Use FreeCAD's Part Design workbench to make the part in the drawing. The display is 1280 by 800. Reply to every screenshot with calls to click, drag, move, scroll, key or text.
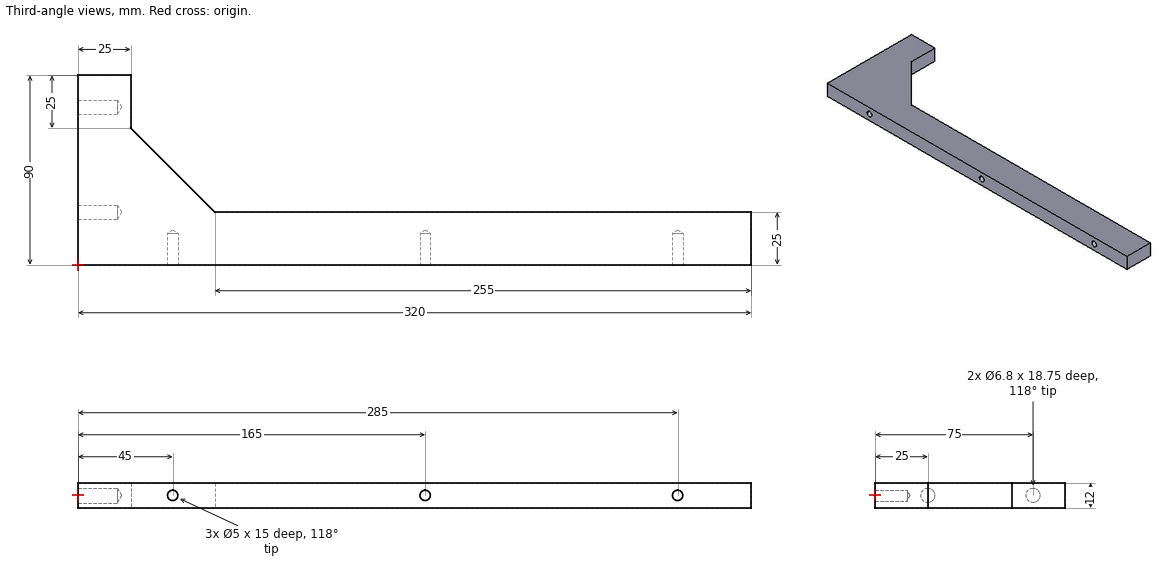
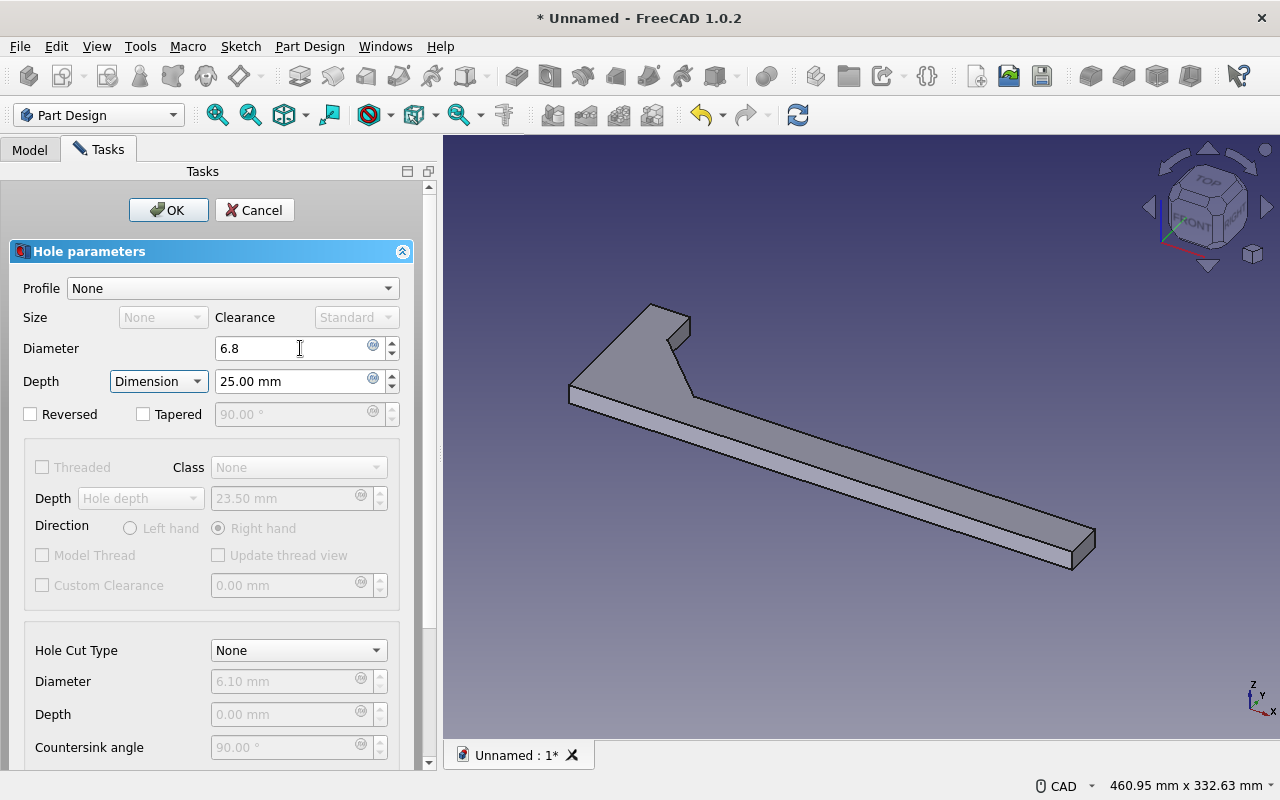
triple_click(300, 382)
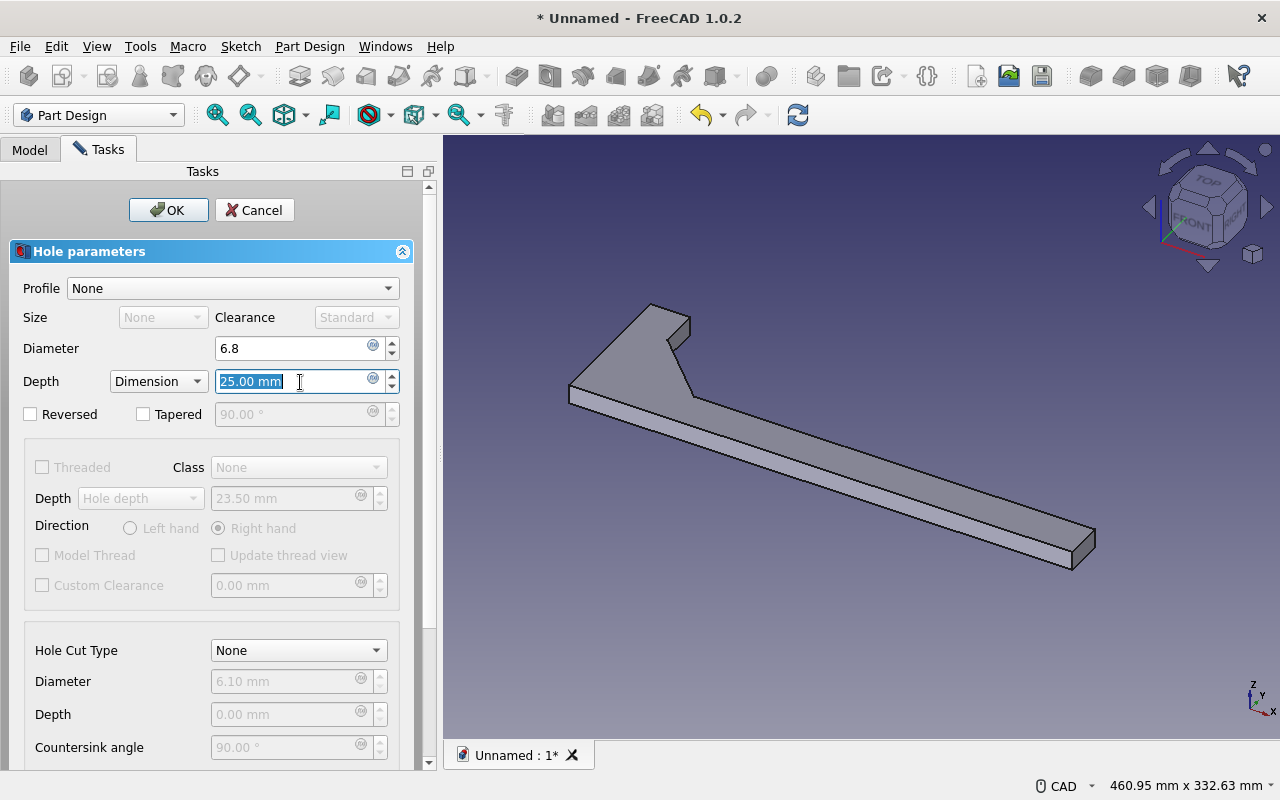
text(18.75)
key(Tab)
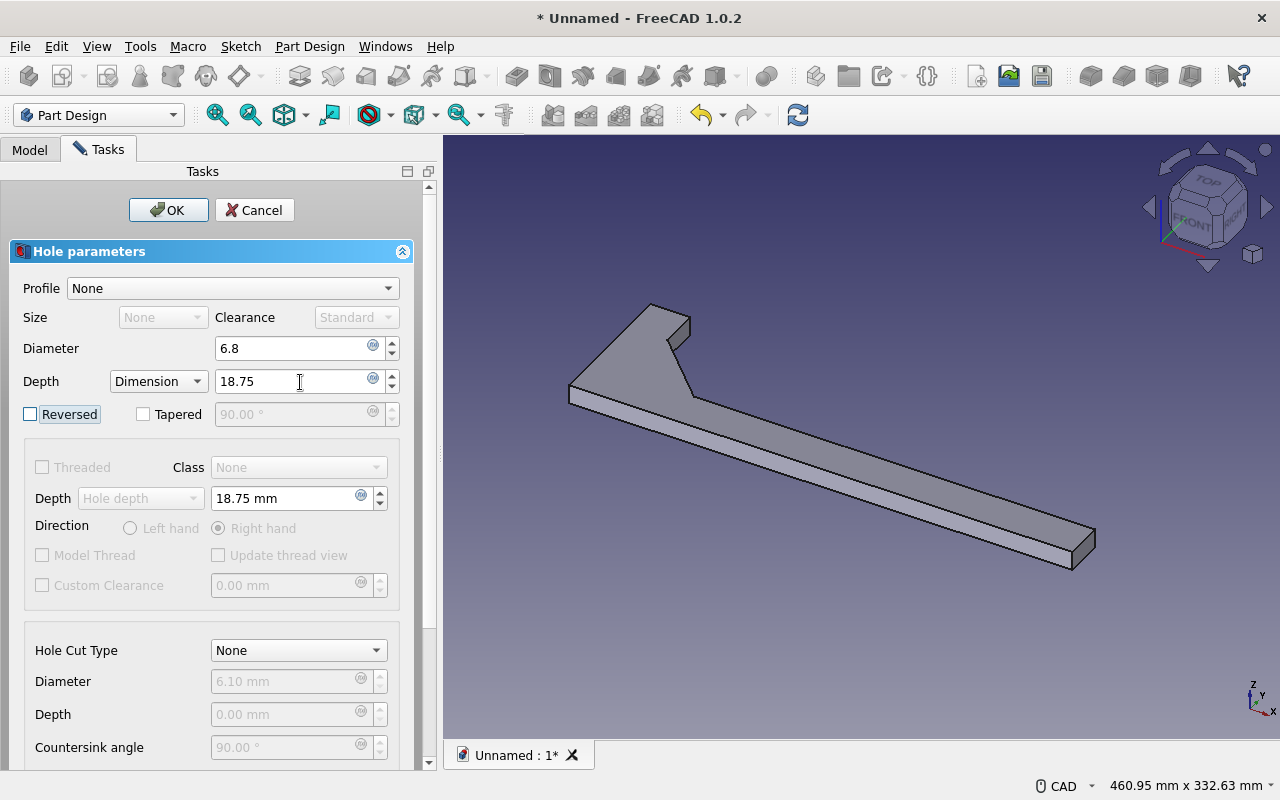
click(31, 414)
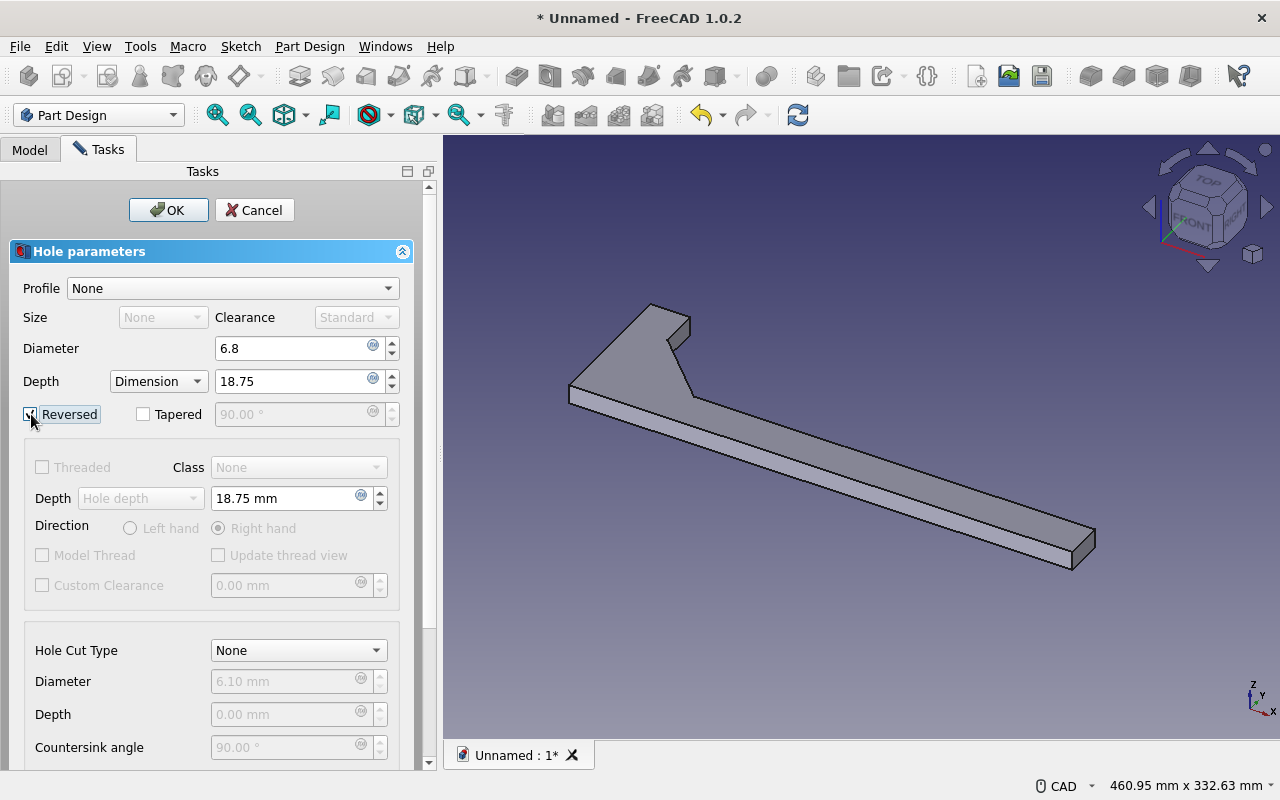
click(169, 210)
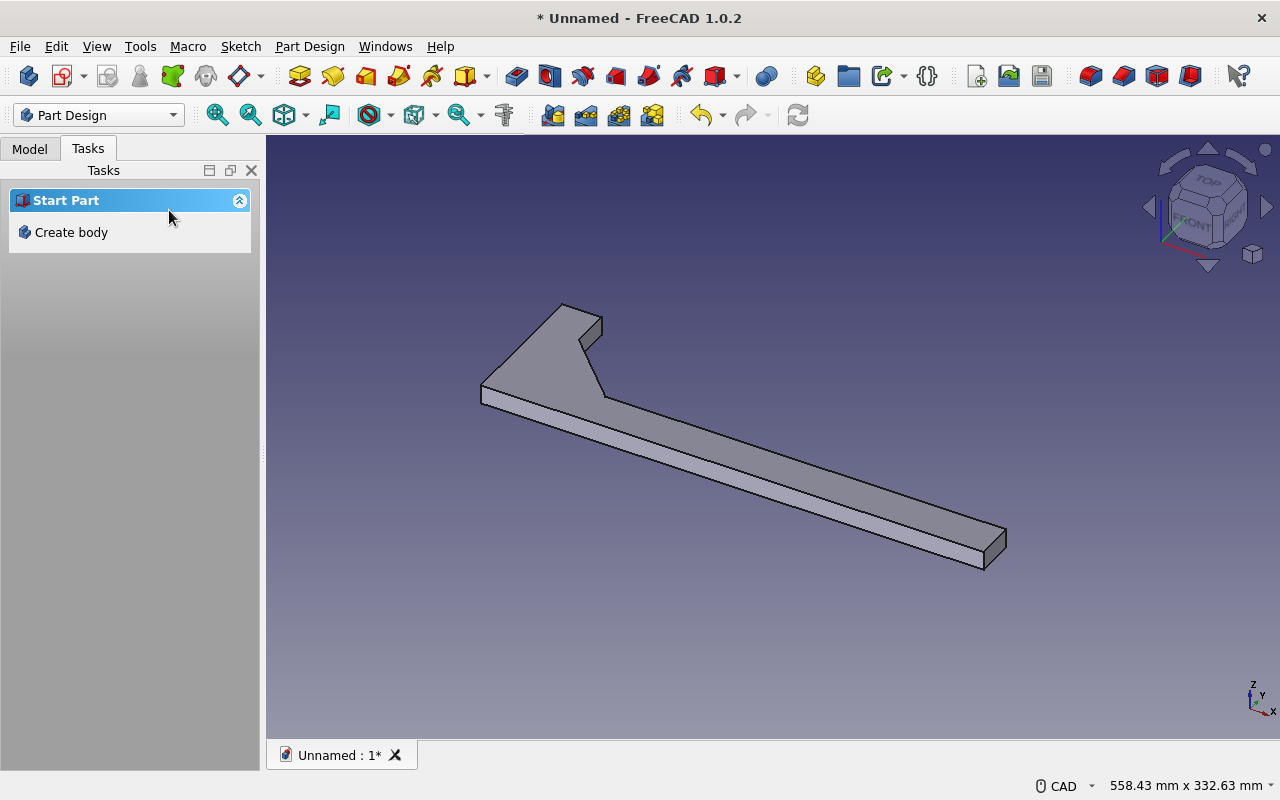
click(62, 76)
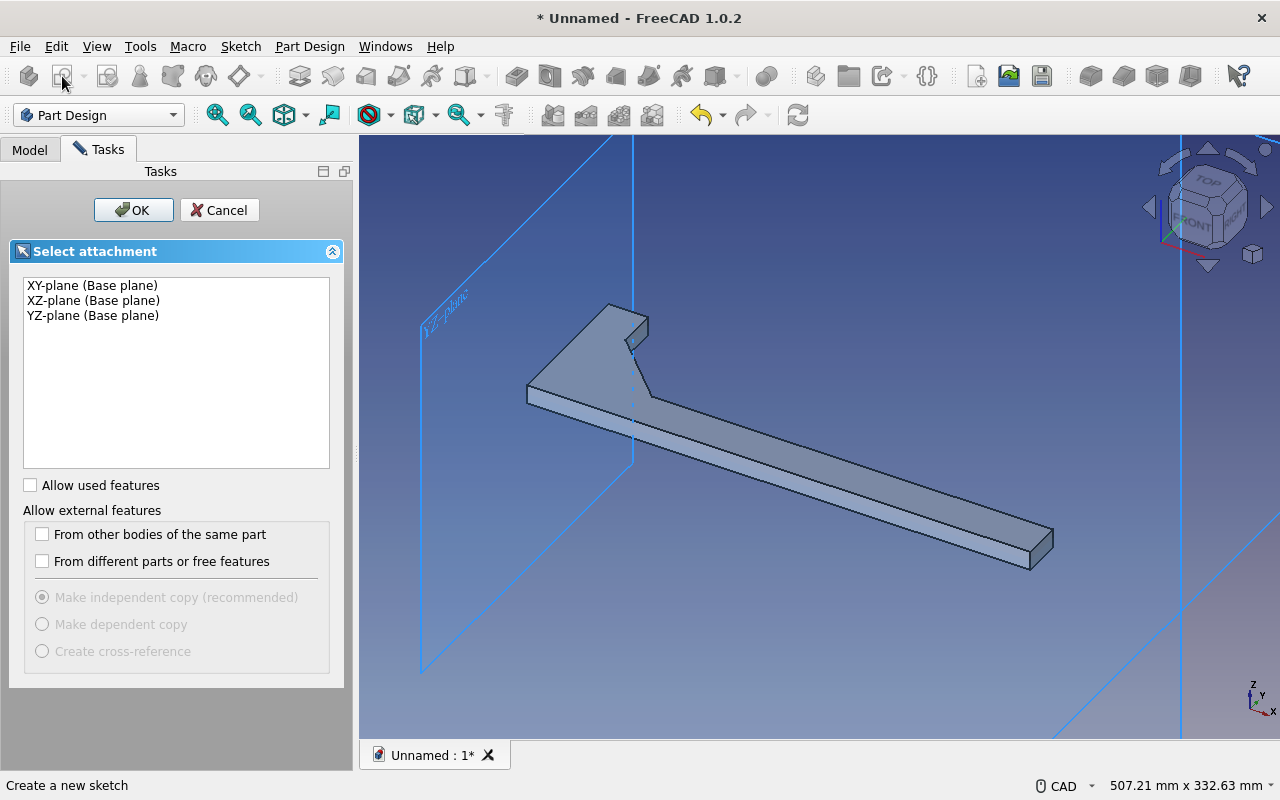
click(84, 300)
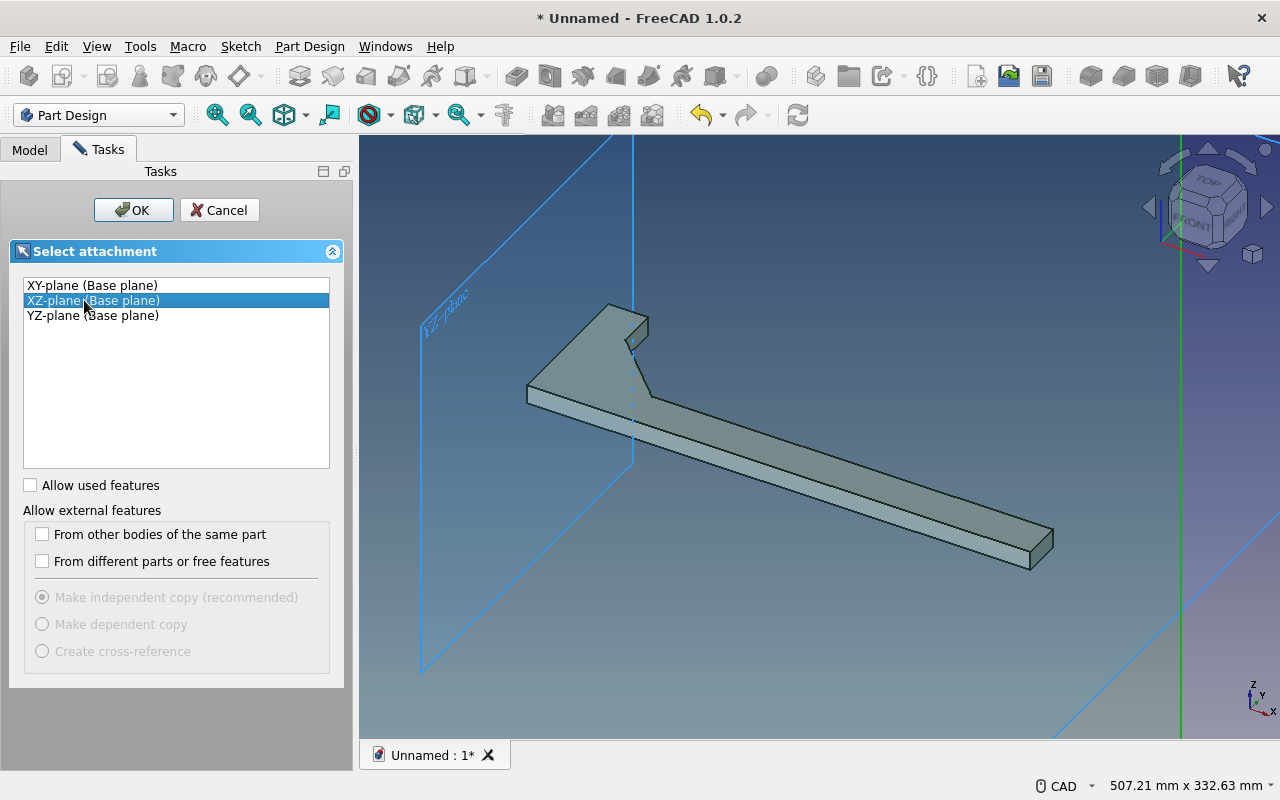
click(134, 210)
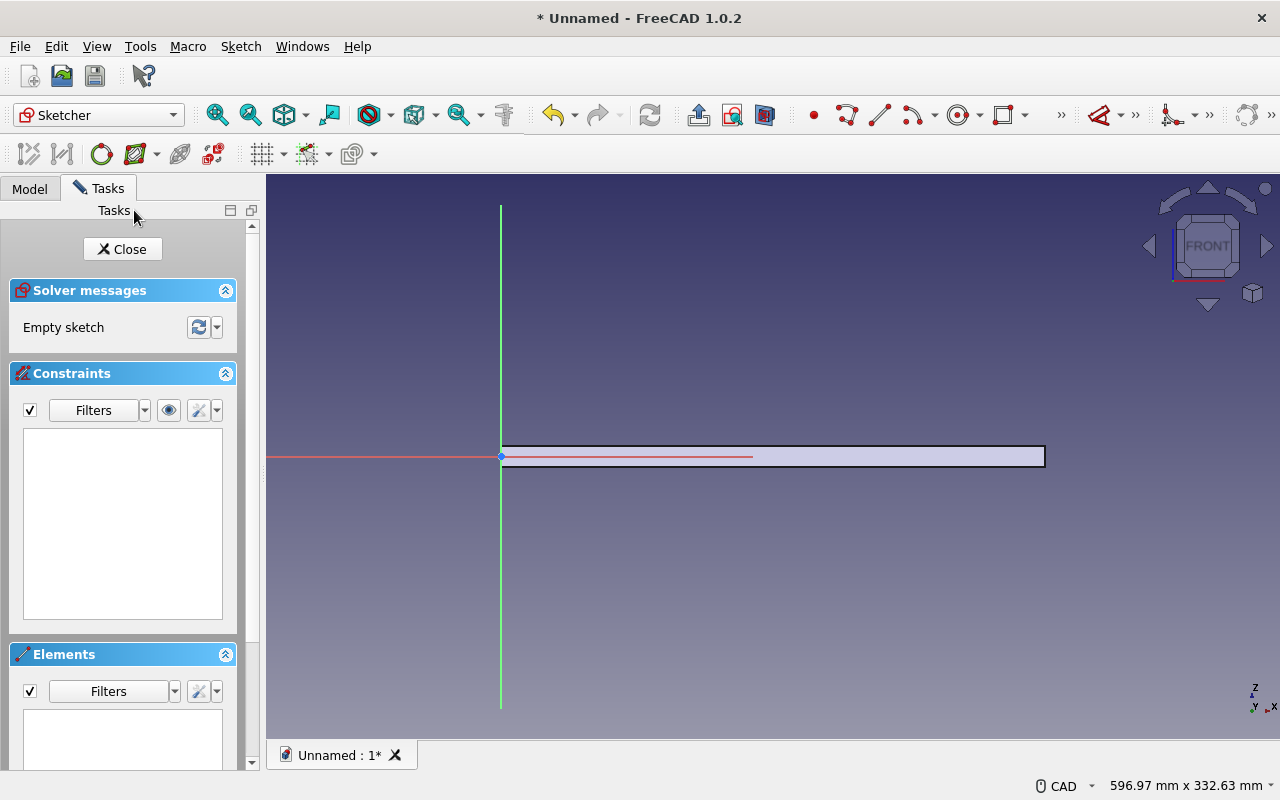
click(958, 116)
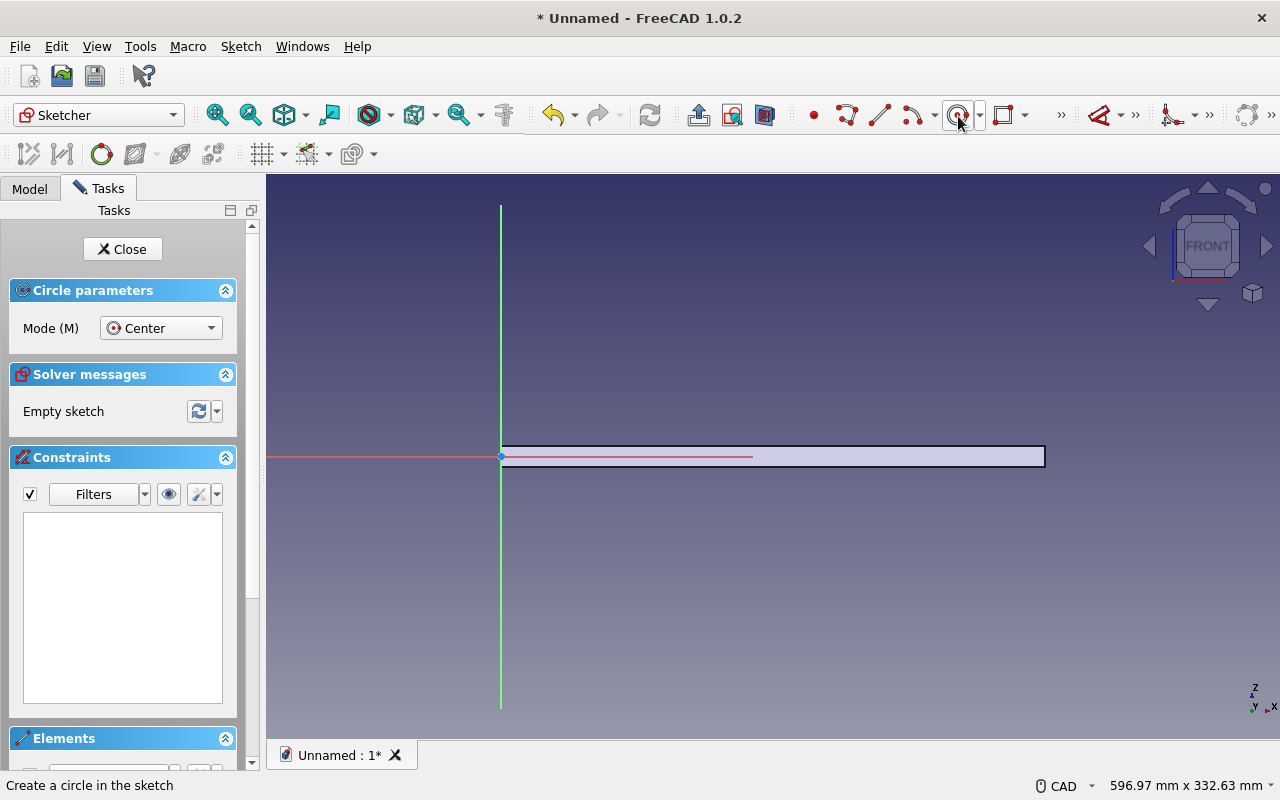
scroll(578, 456, up, 9)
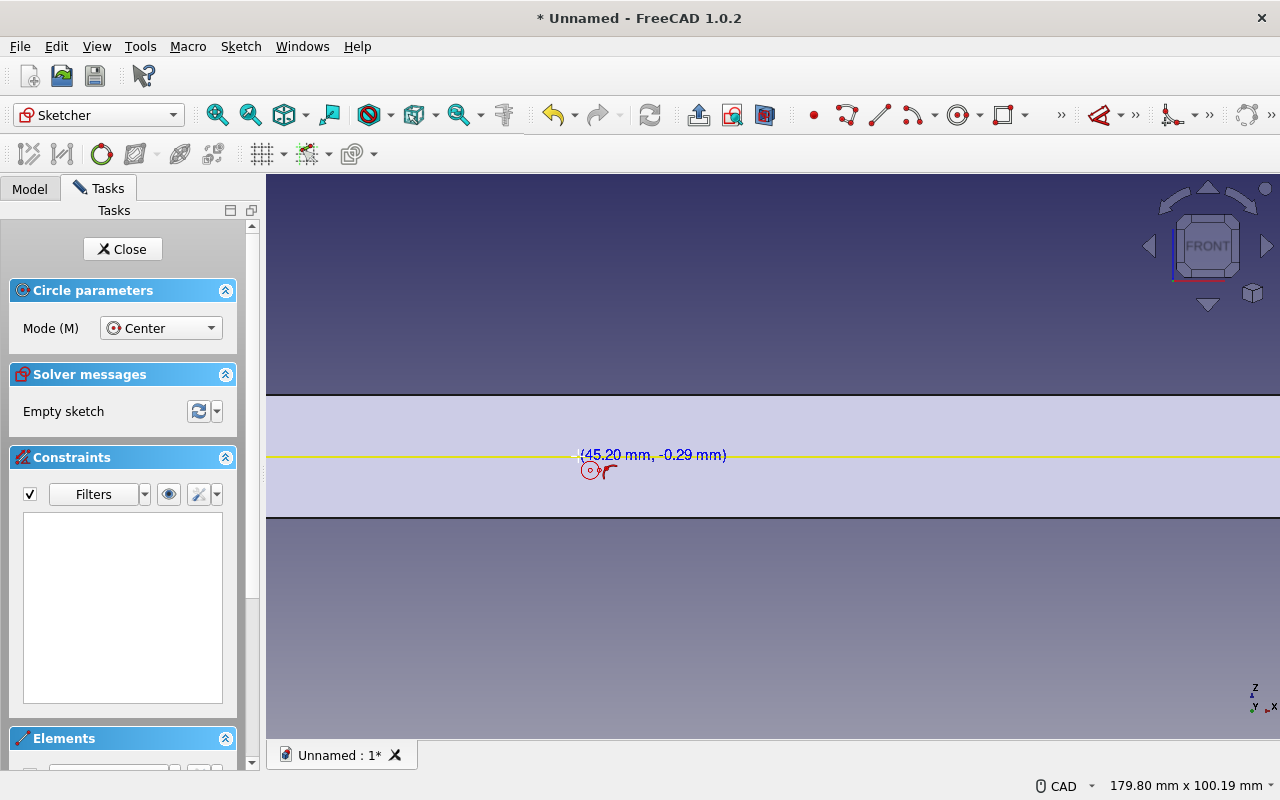
scroll(481, 457, down, 8)